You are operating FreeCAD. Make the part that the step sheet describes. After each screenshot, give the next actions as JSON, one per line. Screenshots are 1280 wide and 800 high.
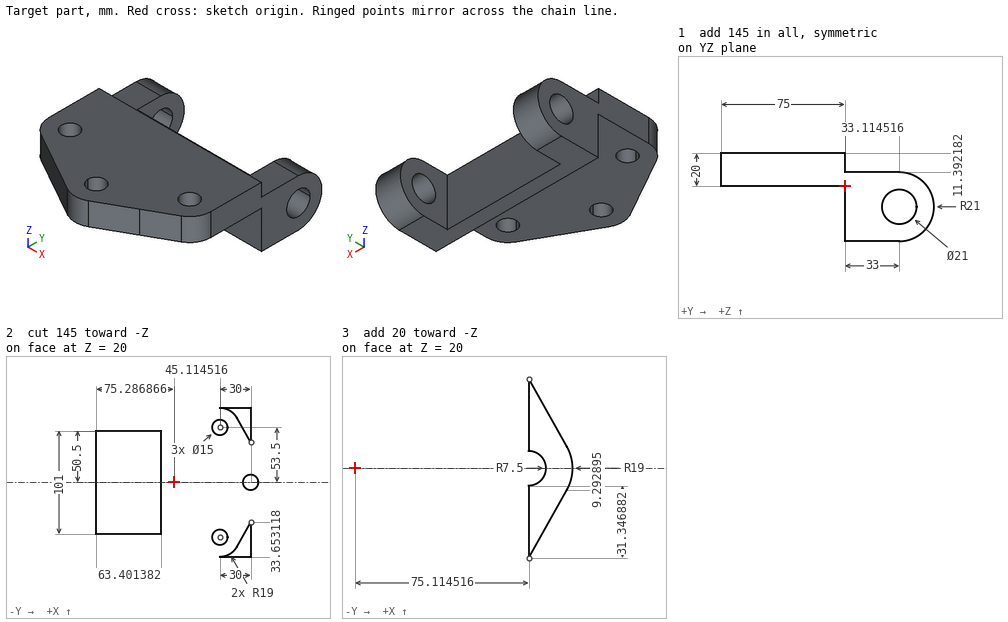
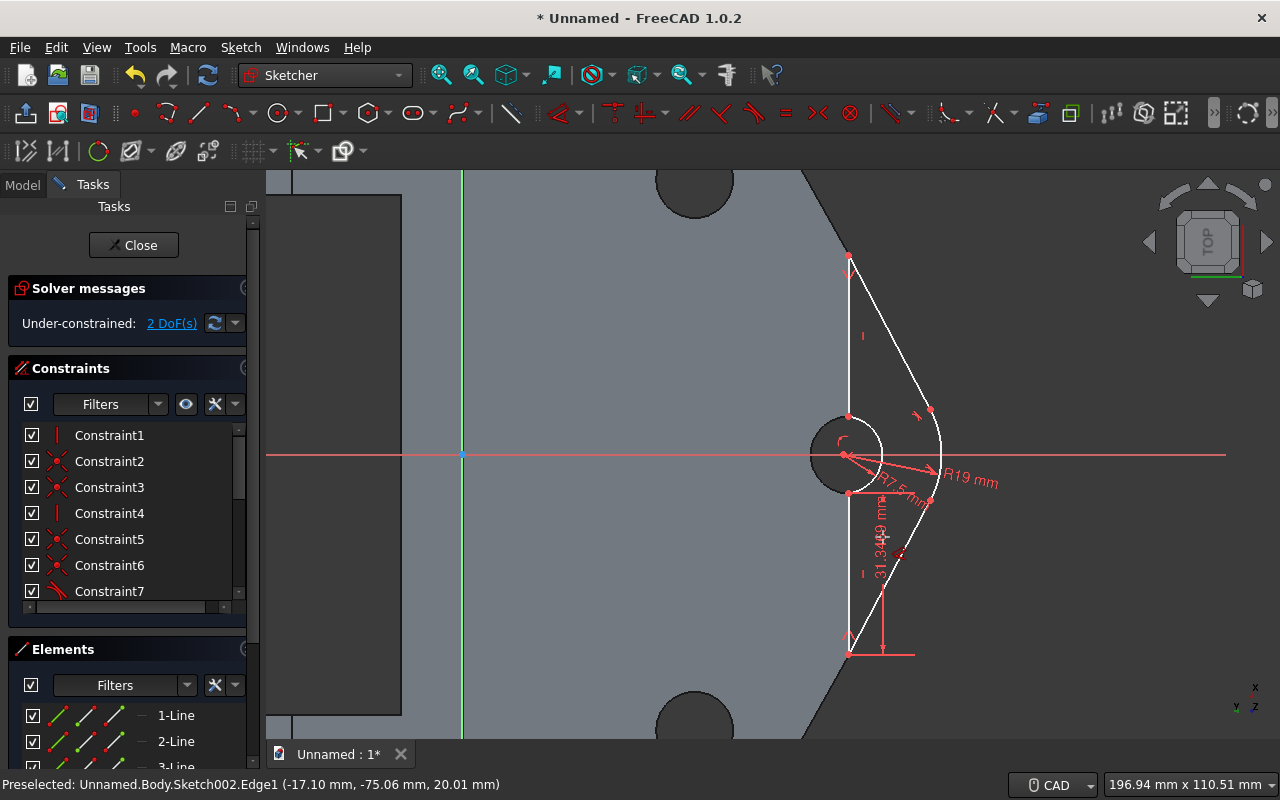
{"action": "left_click", "coordinate": [930, 501]}
{"action": "left_click", "coordinate": [428, 478]}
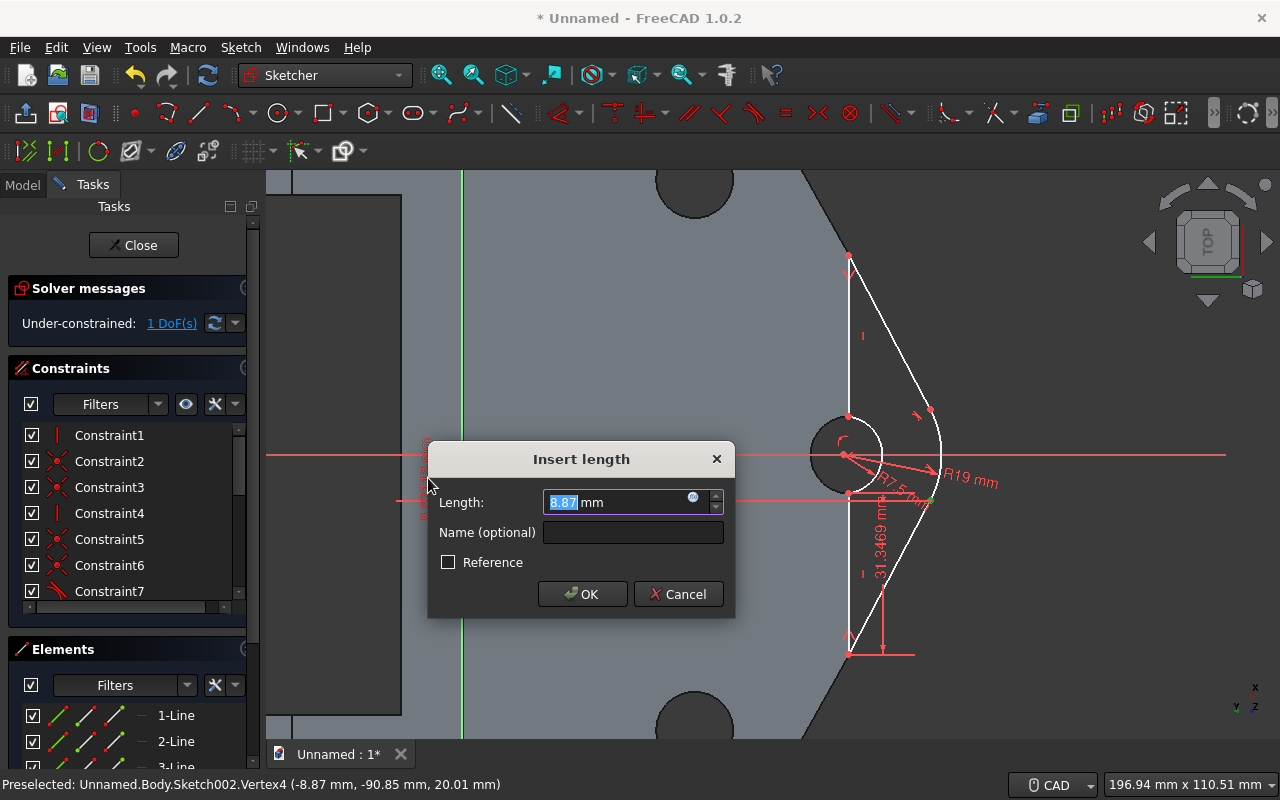
{"action": "type", "text": "9.292895"}
{"action": "key", "text": "Return"}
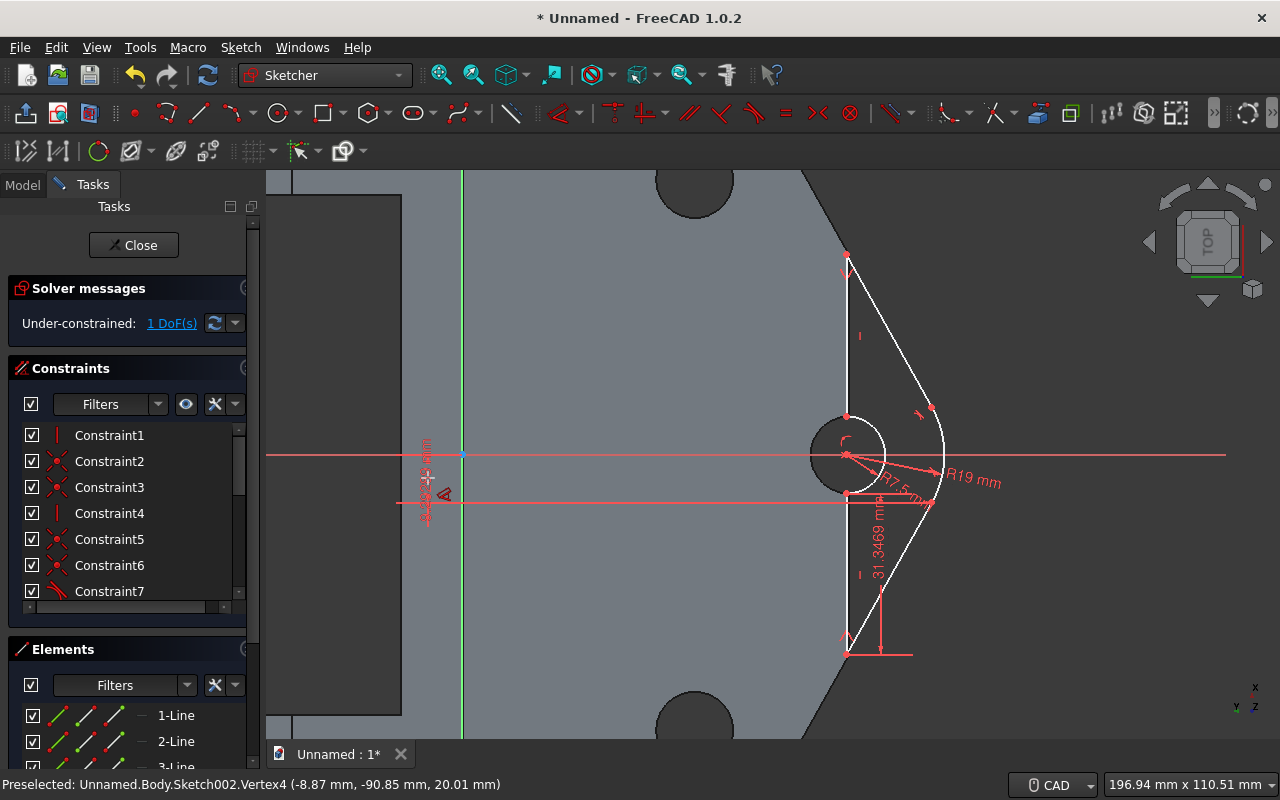
{"action": "left_click", "coordinate": [847, 494]}
{"action": "left_click", "coordinate": [654, 528]}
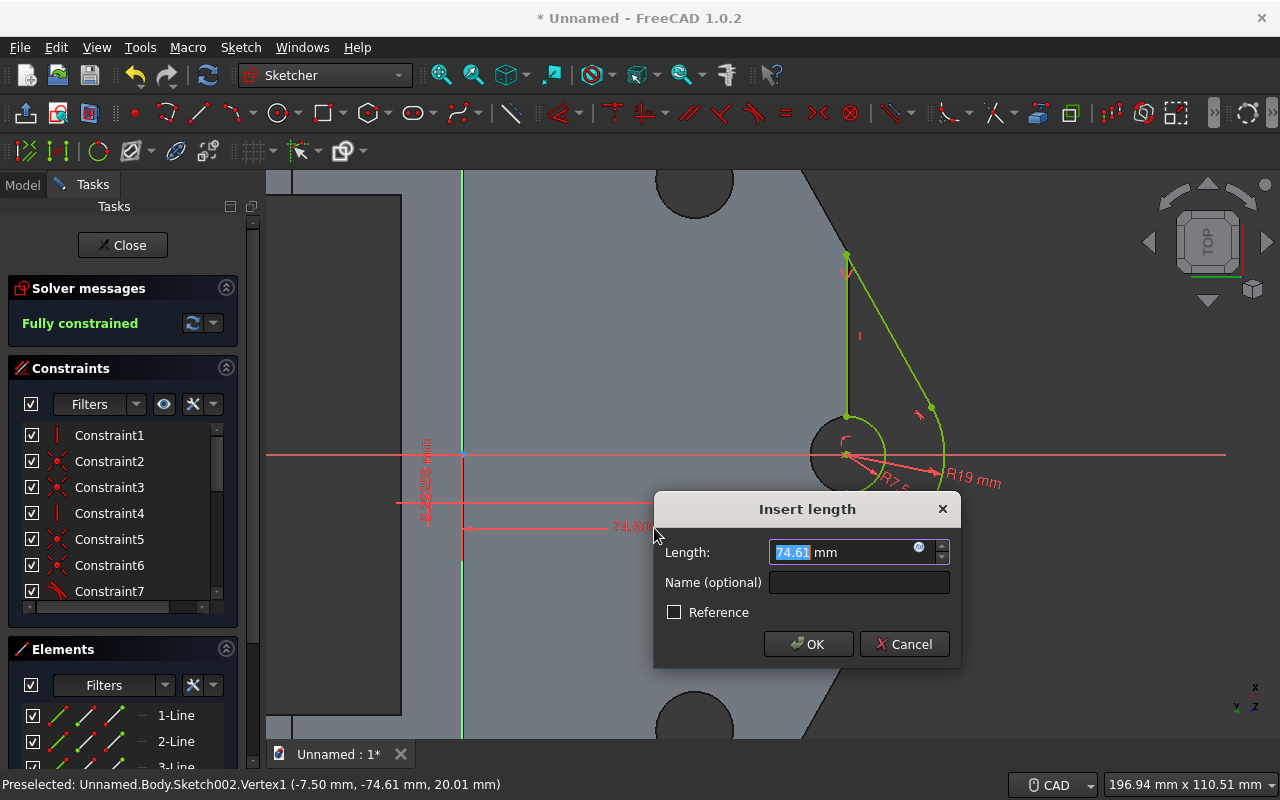
{"action": "type", "text": "75.114516"}
{"action": "key", "text": "Return"}
{"action": "key", "text": "Escape"}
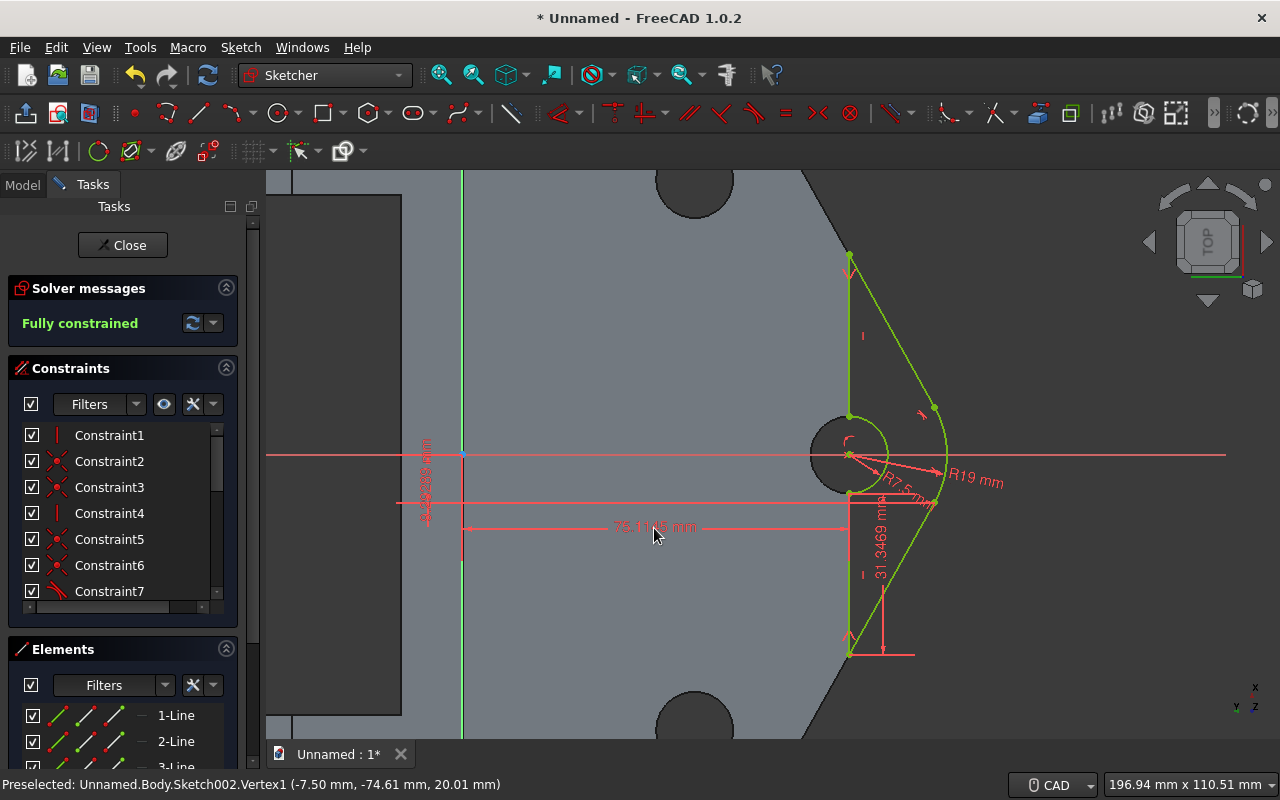
{"action": "left_click", "coordinate": [123, 245]}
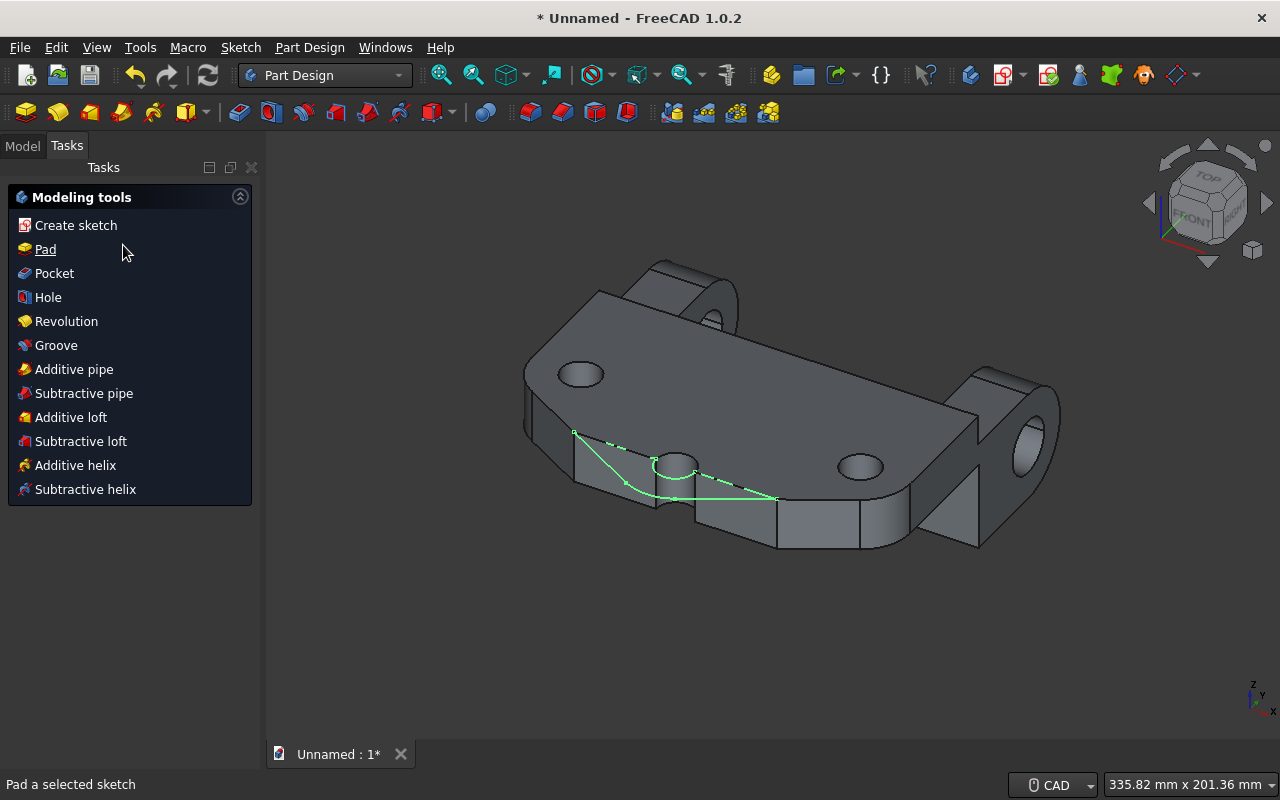
{"action": "left_click", "coordinate": [26, 112]}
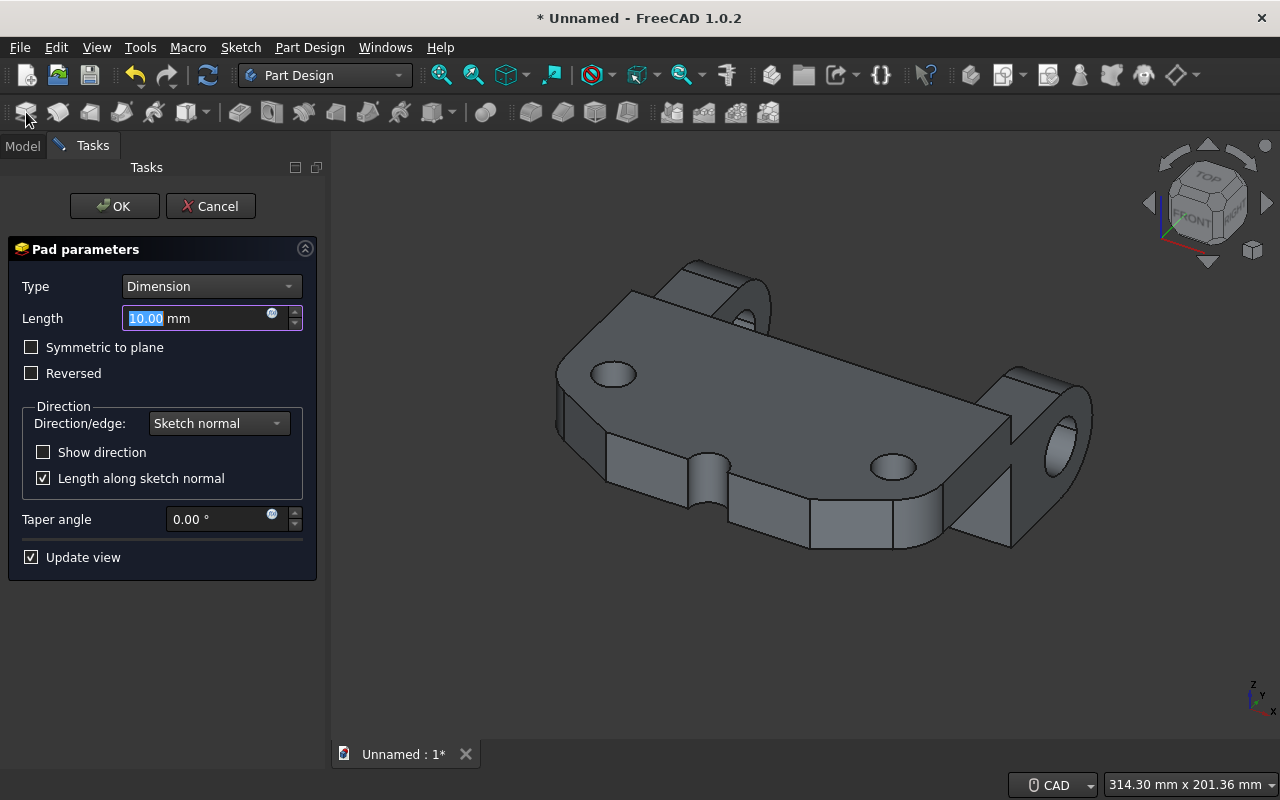
{"action": "type", "text": "20"}
{"action": "key", "text": "Tab"}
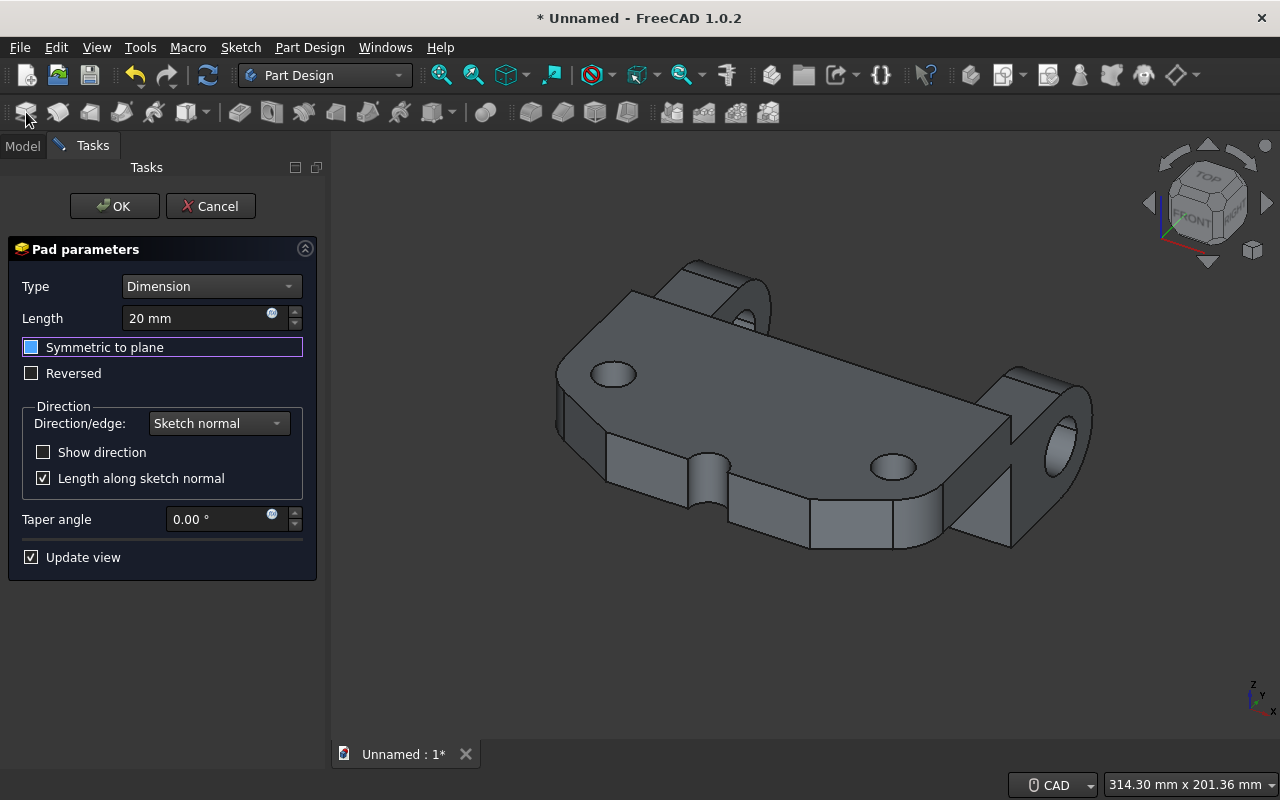
{"action": "left_click", "coordinate": [30, 373]}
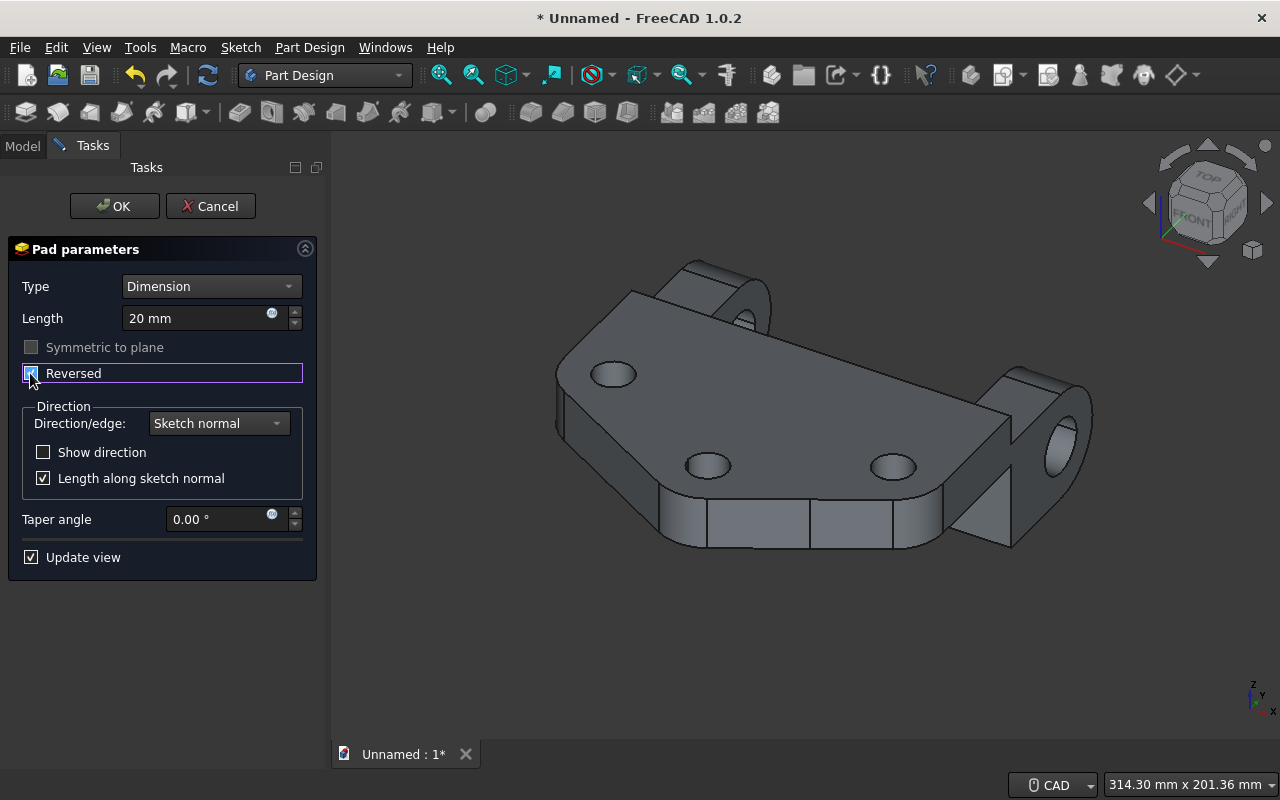
{"action": "left_click", "coordinate": [115, 206]}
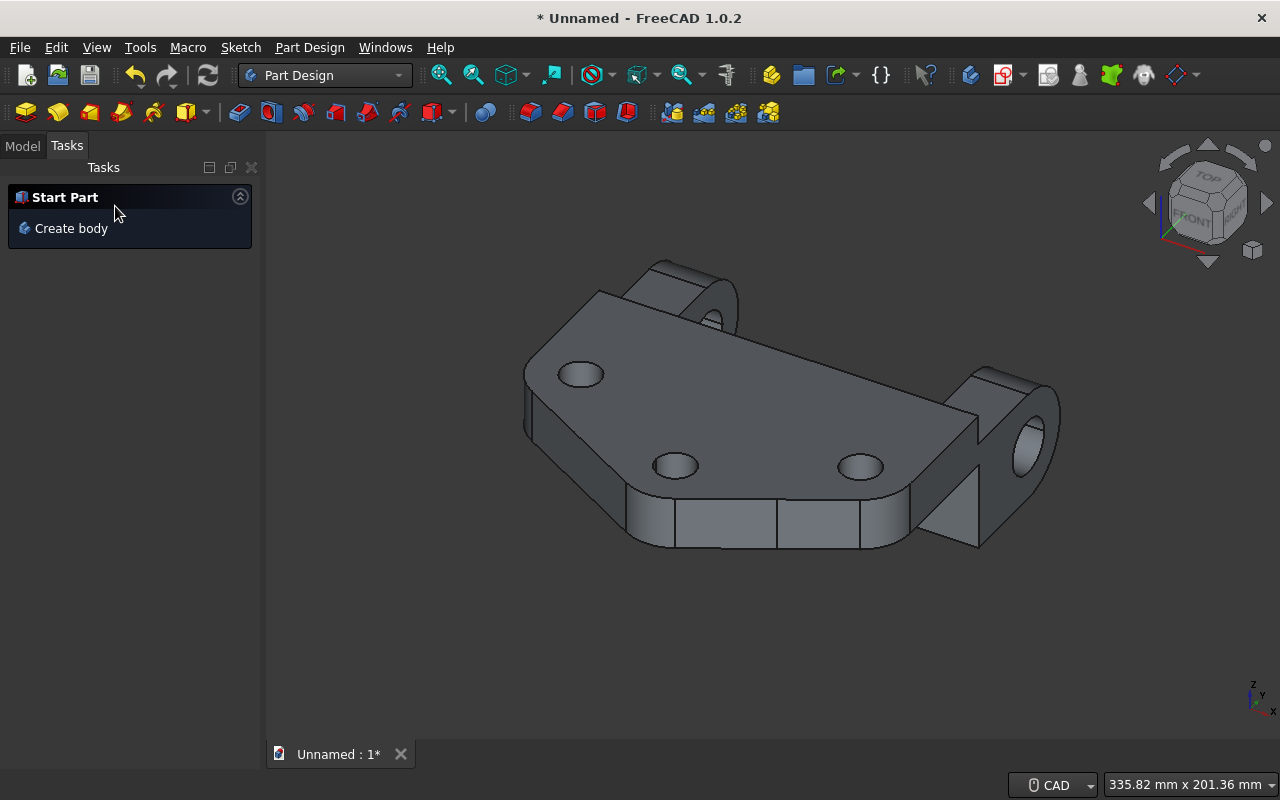
{"action": "key", "text": "0"}